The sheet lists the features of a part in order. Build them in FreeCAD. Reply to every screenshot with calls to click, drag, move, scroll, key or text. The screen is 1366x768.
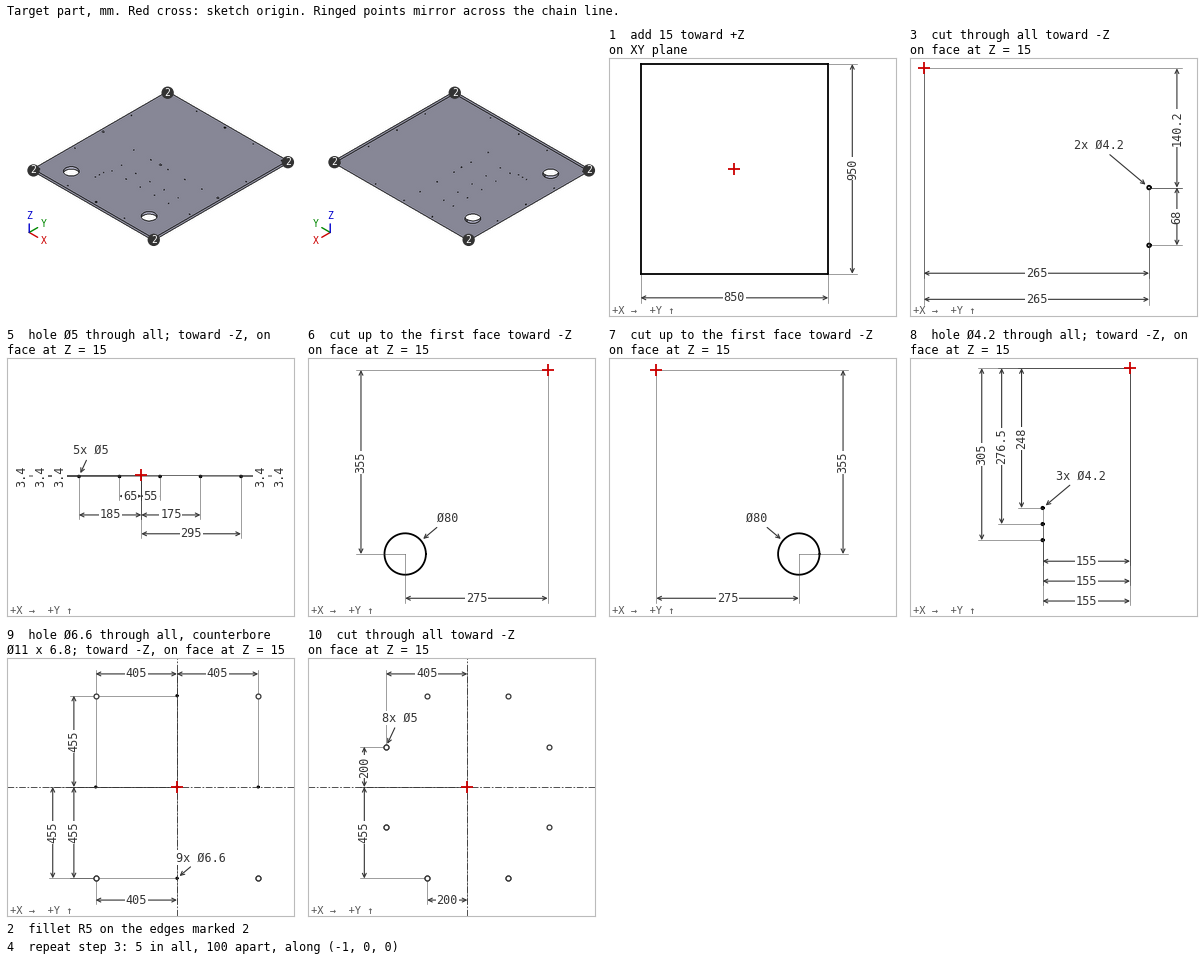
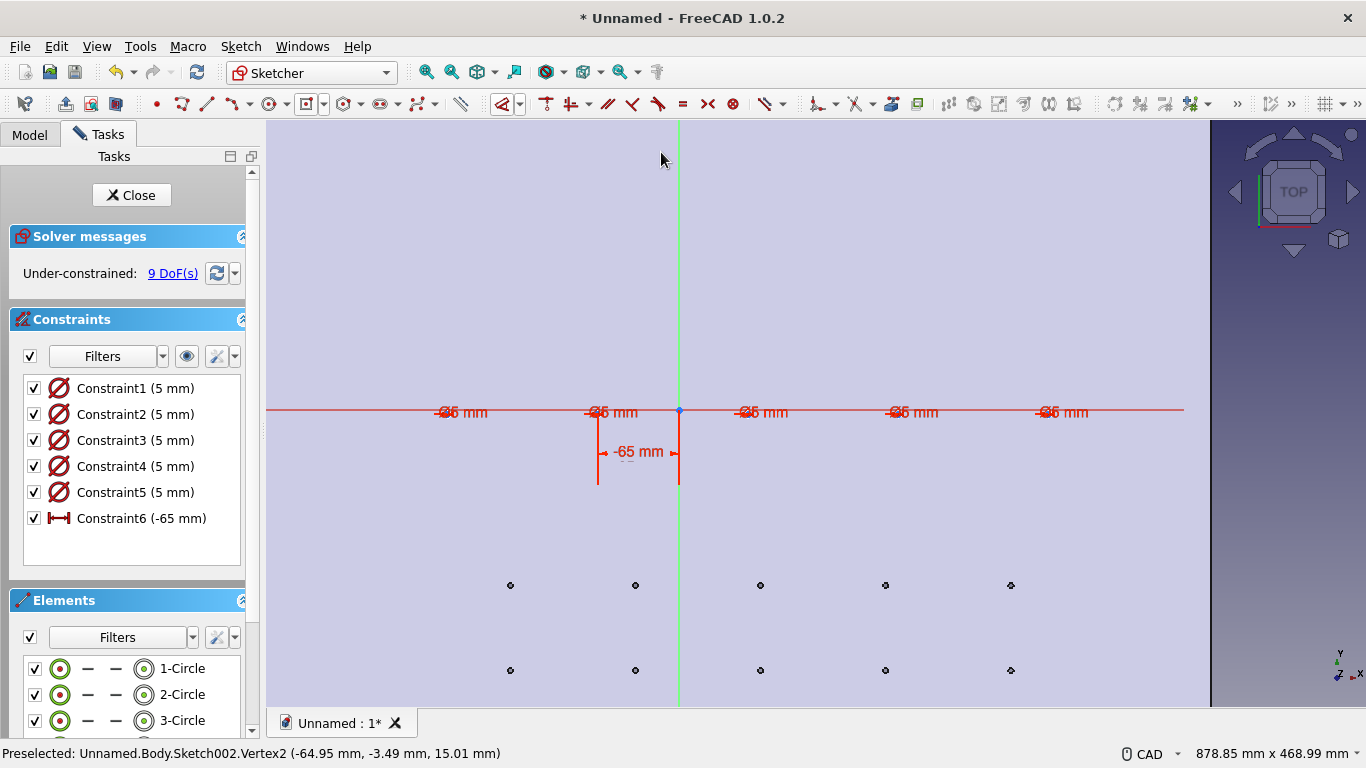
click(748, 414)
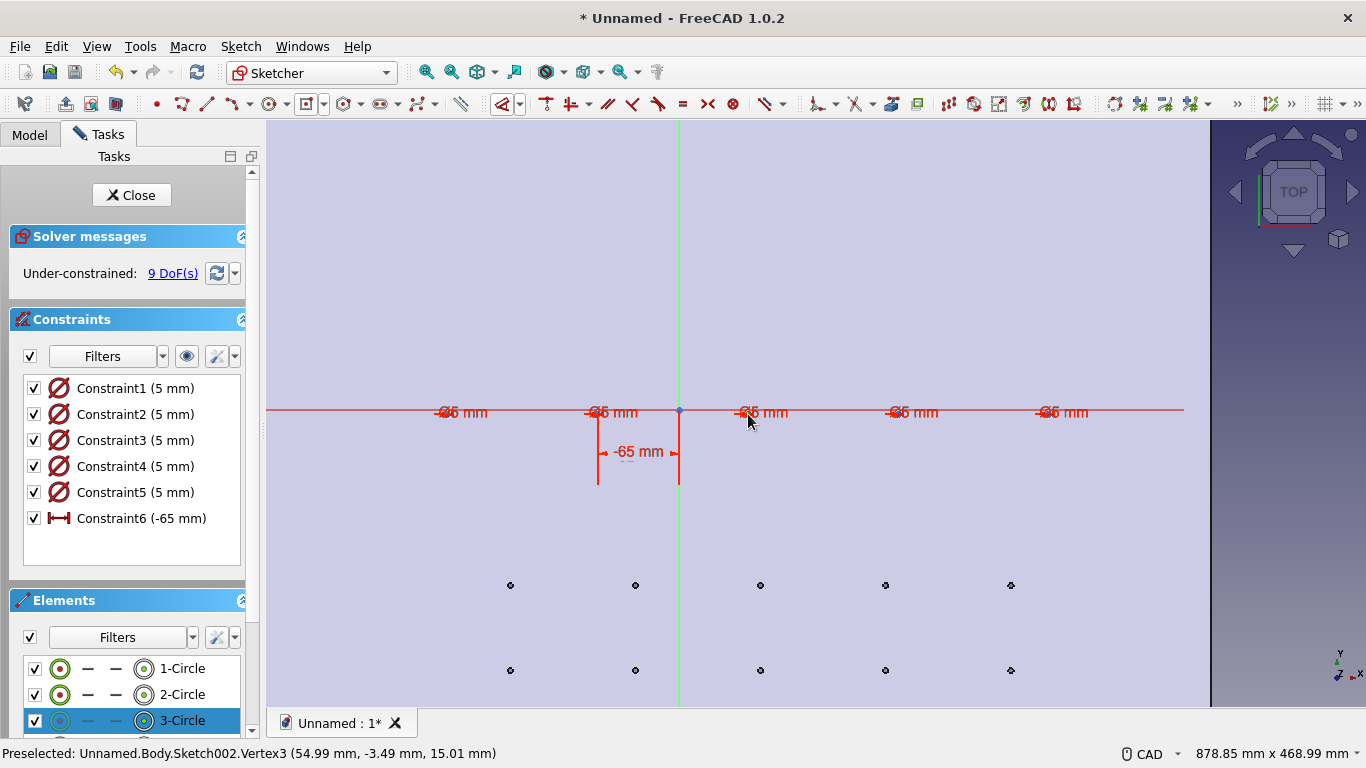
key(l)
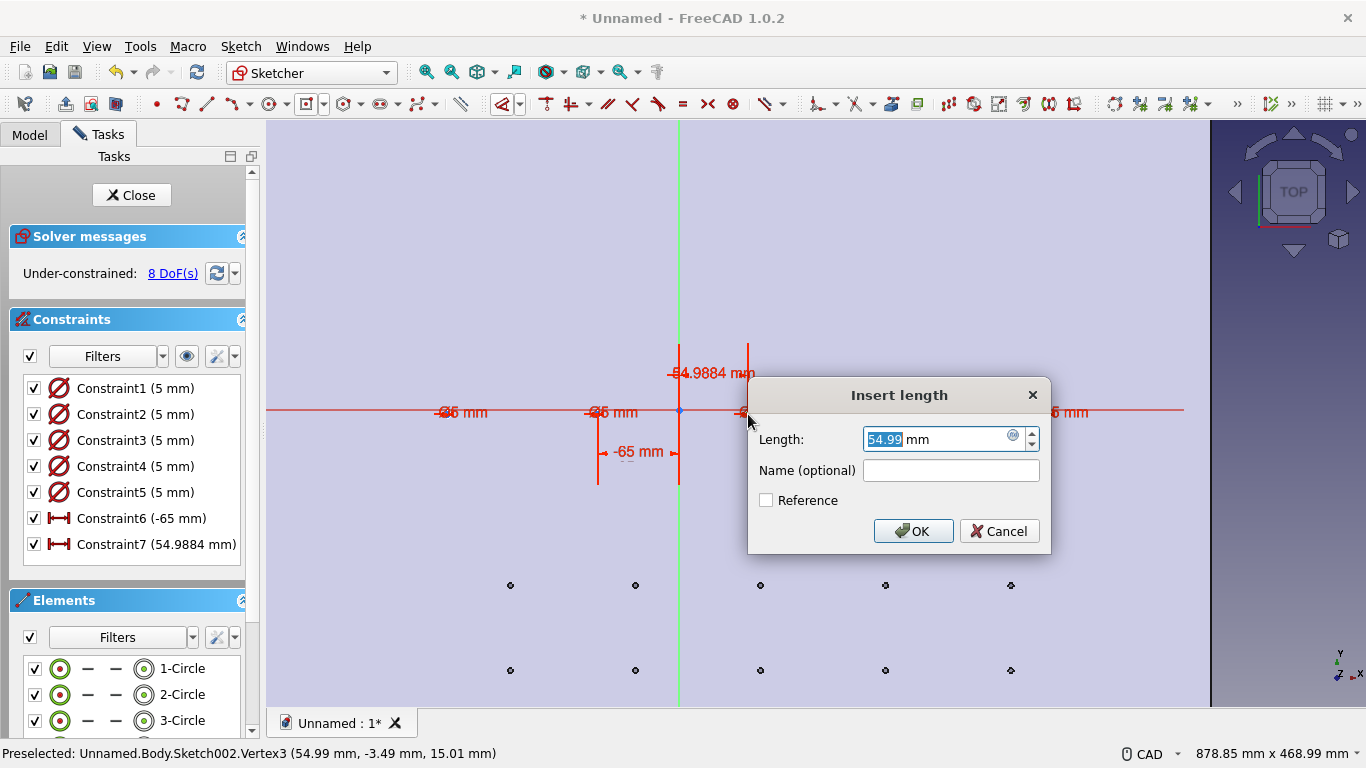
text(55)
key(Return)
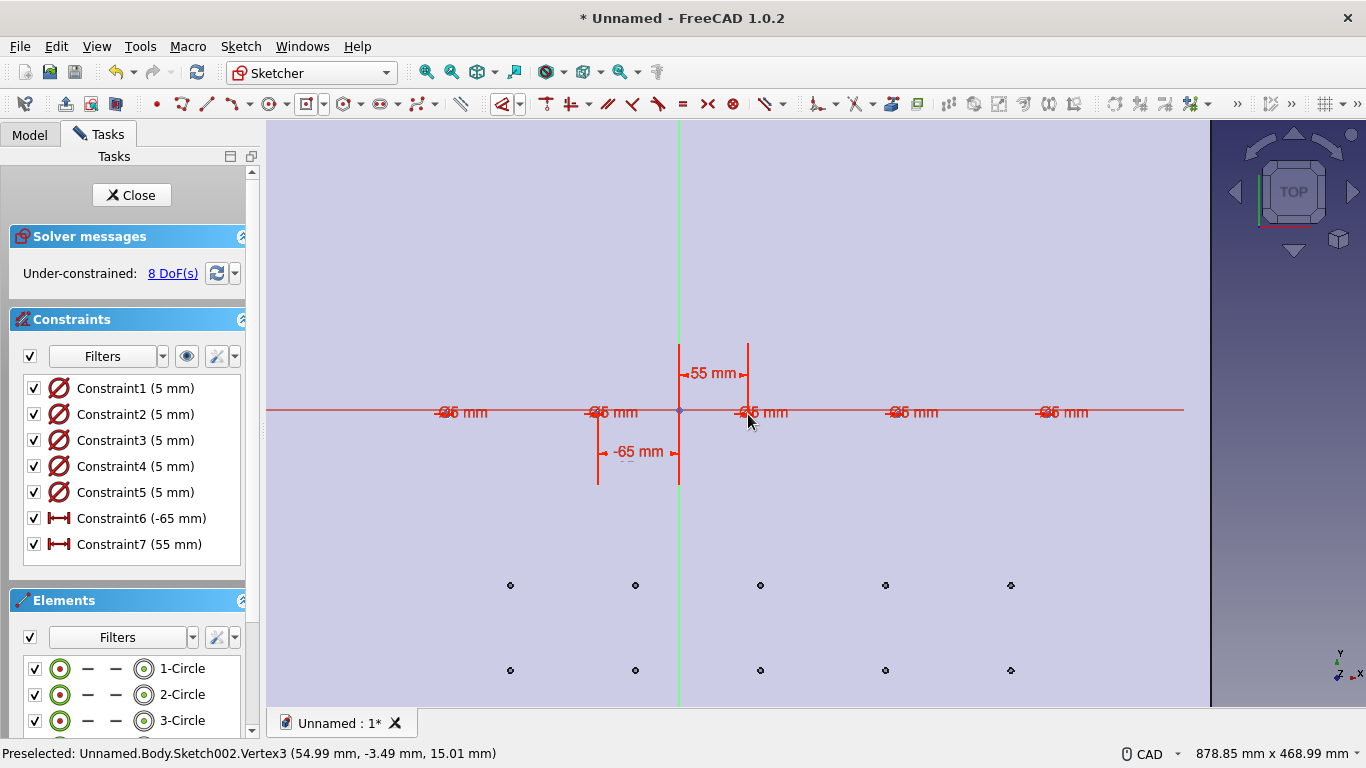
click(448, 414)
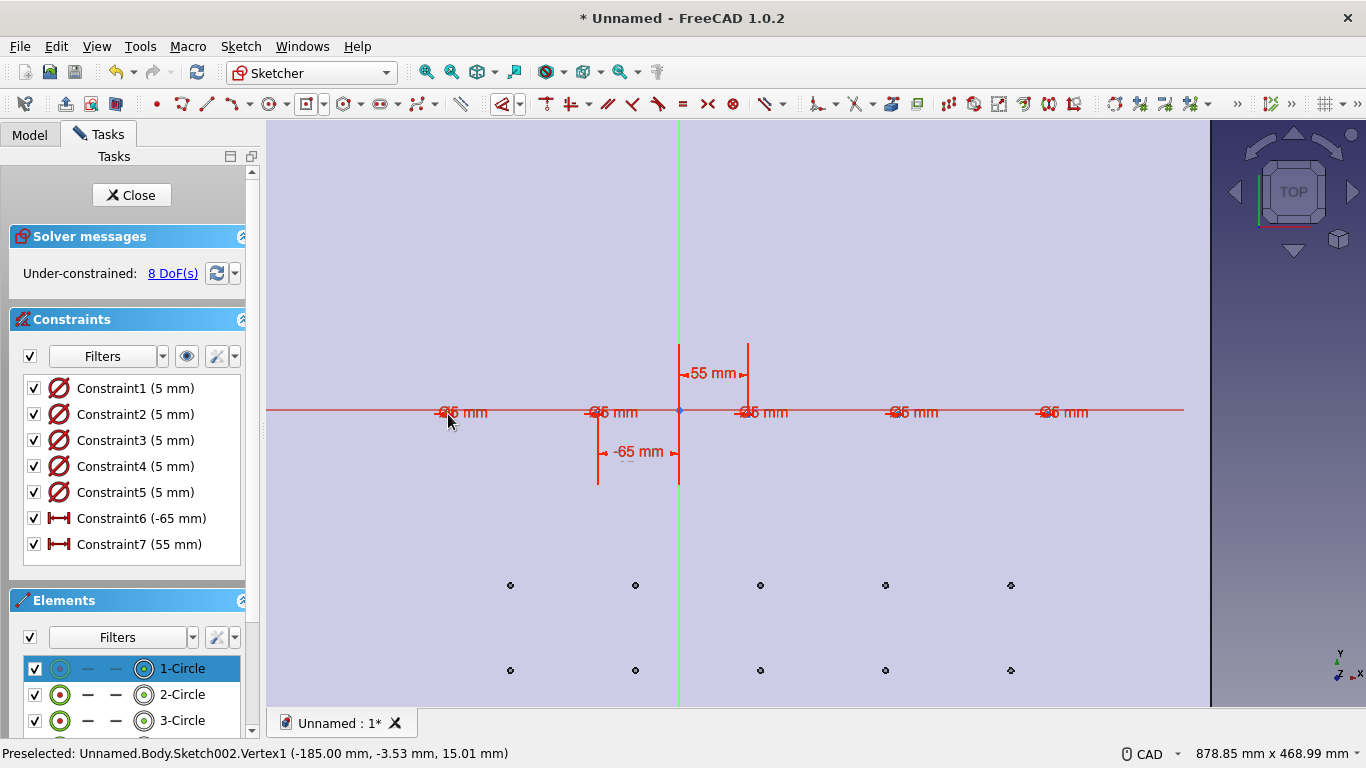
click(520, 104)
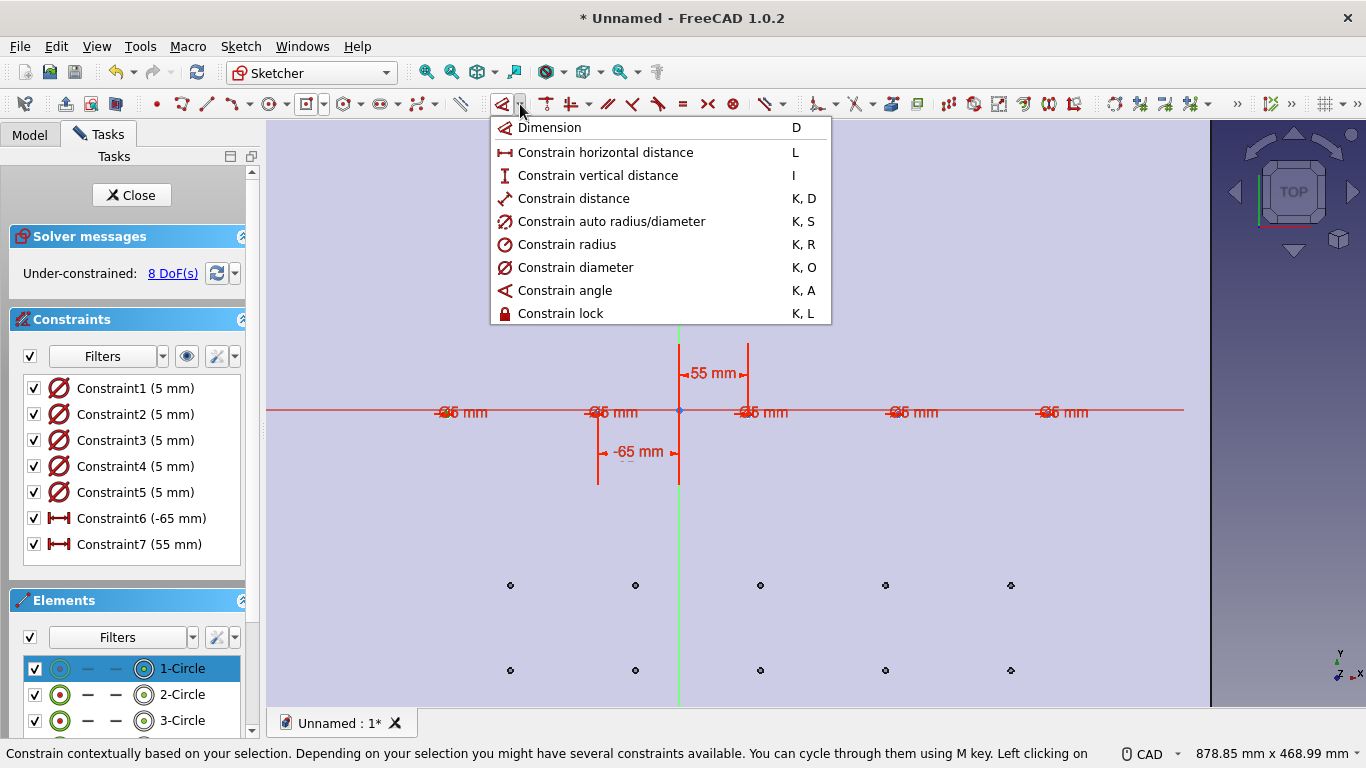
click(661, 152)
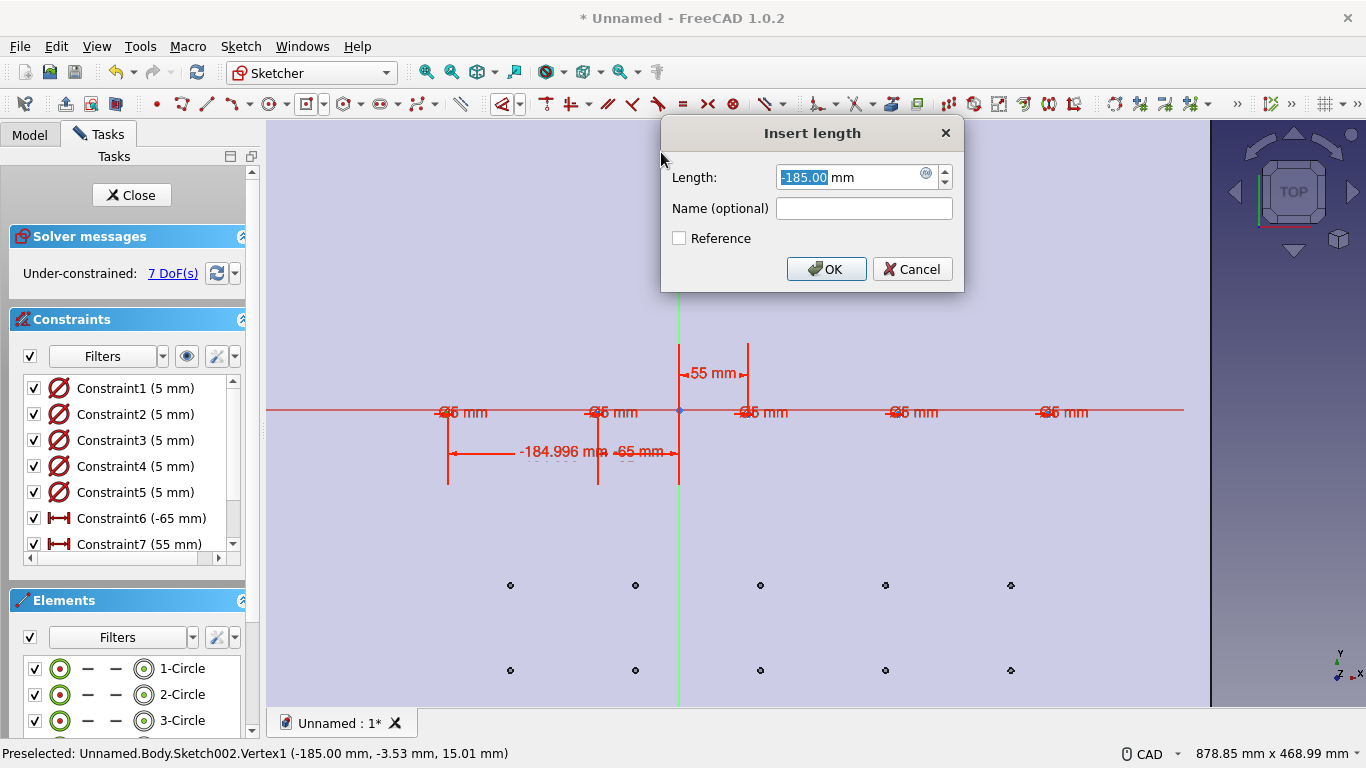
text(-185)
key(Return)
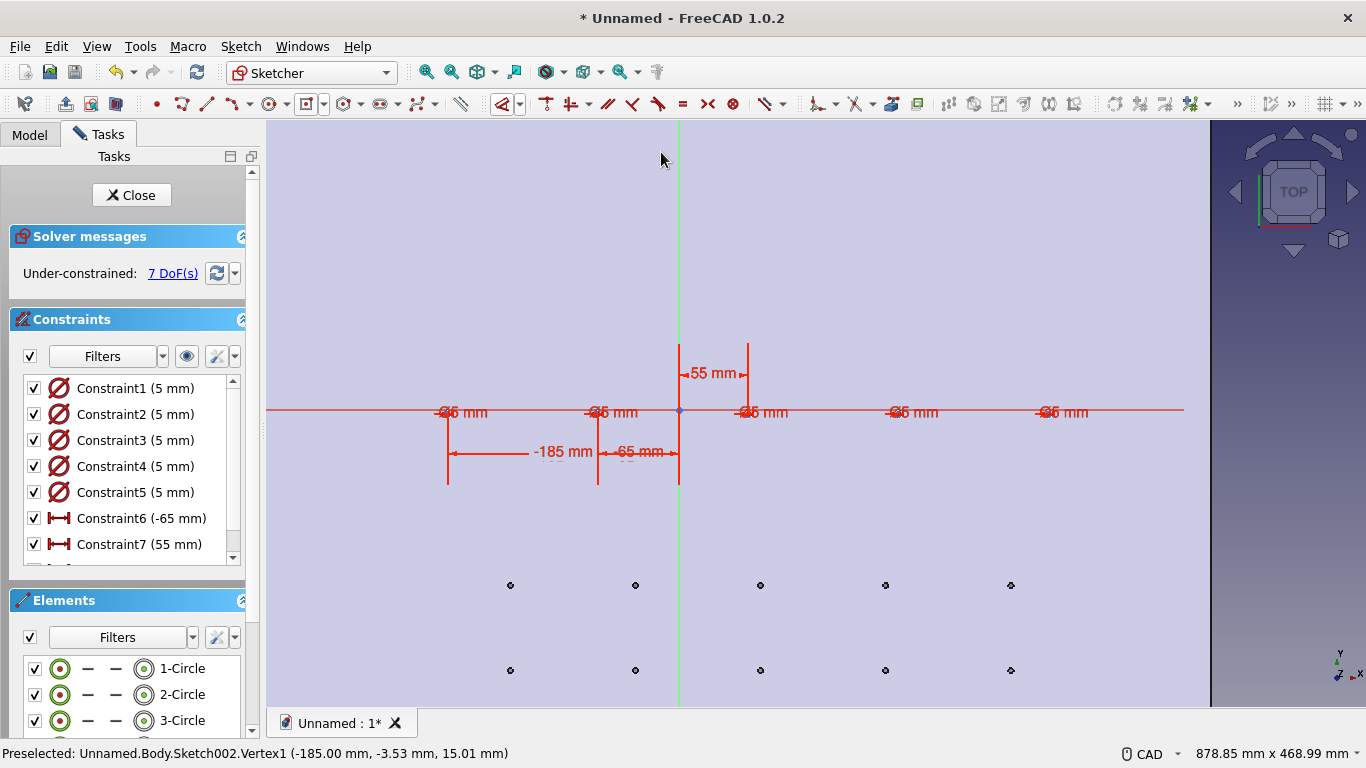
scroll(448, 414, up, 12)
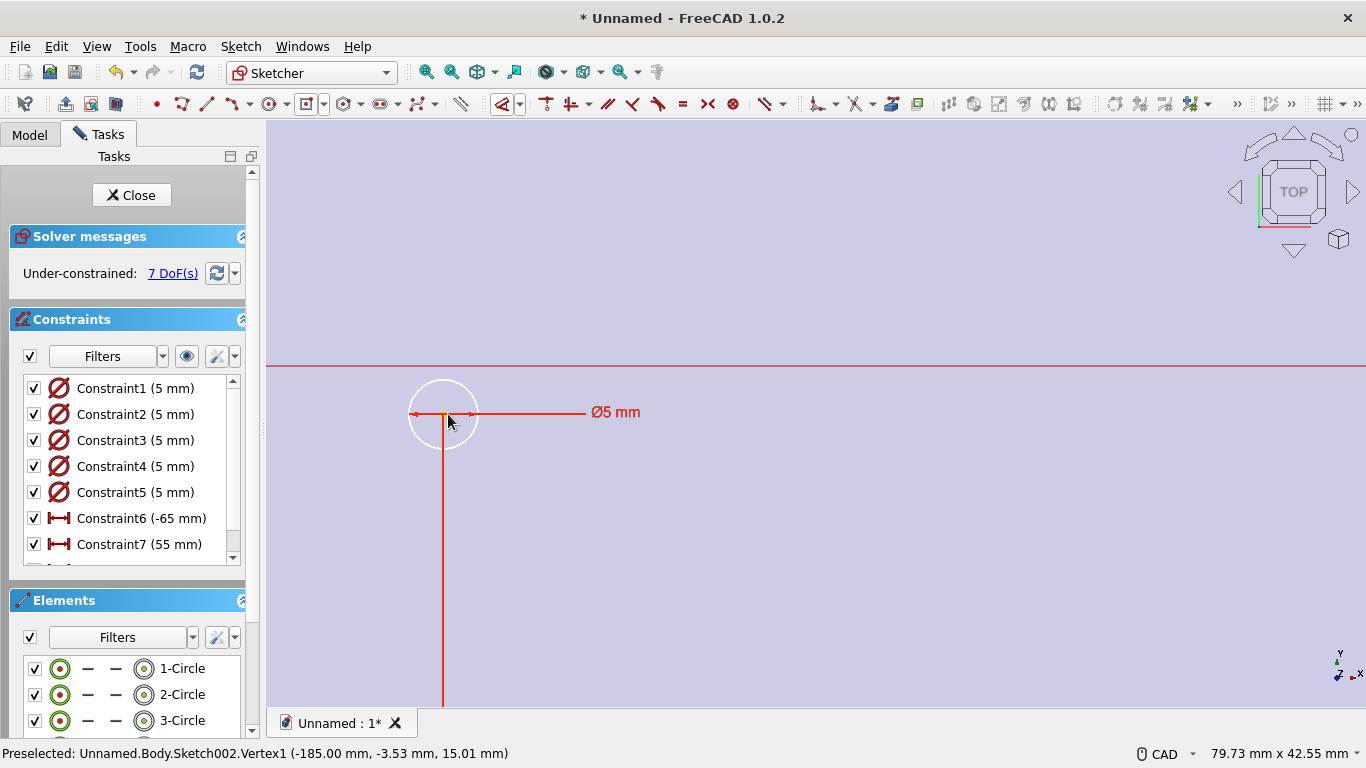
click(443, 414)